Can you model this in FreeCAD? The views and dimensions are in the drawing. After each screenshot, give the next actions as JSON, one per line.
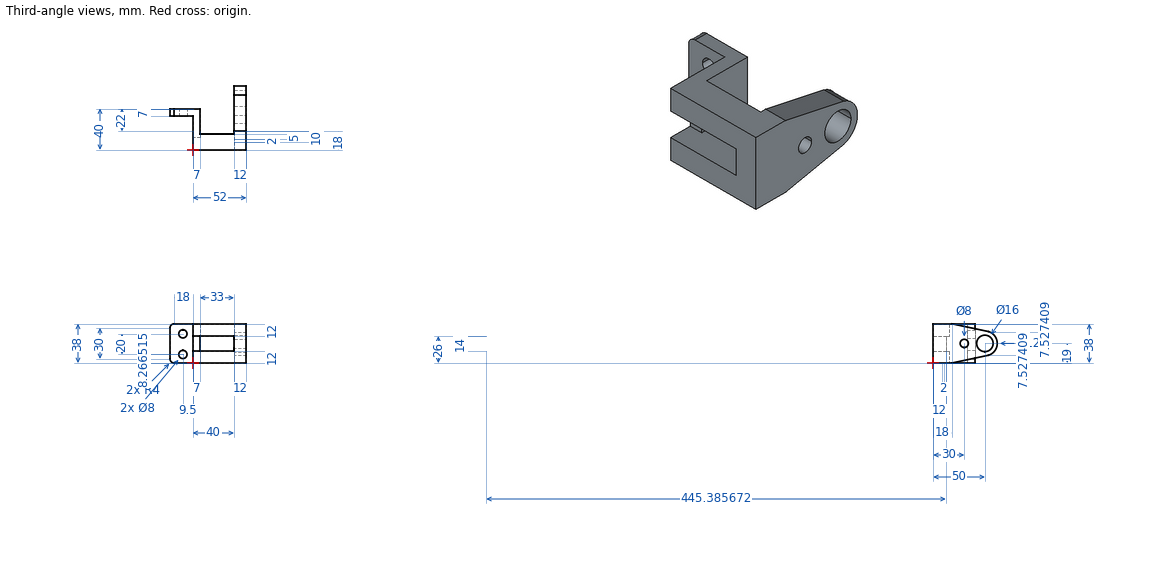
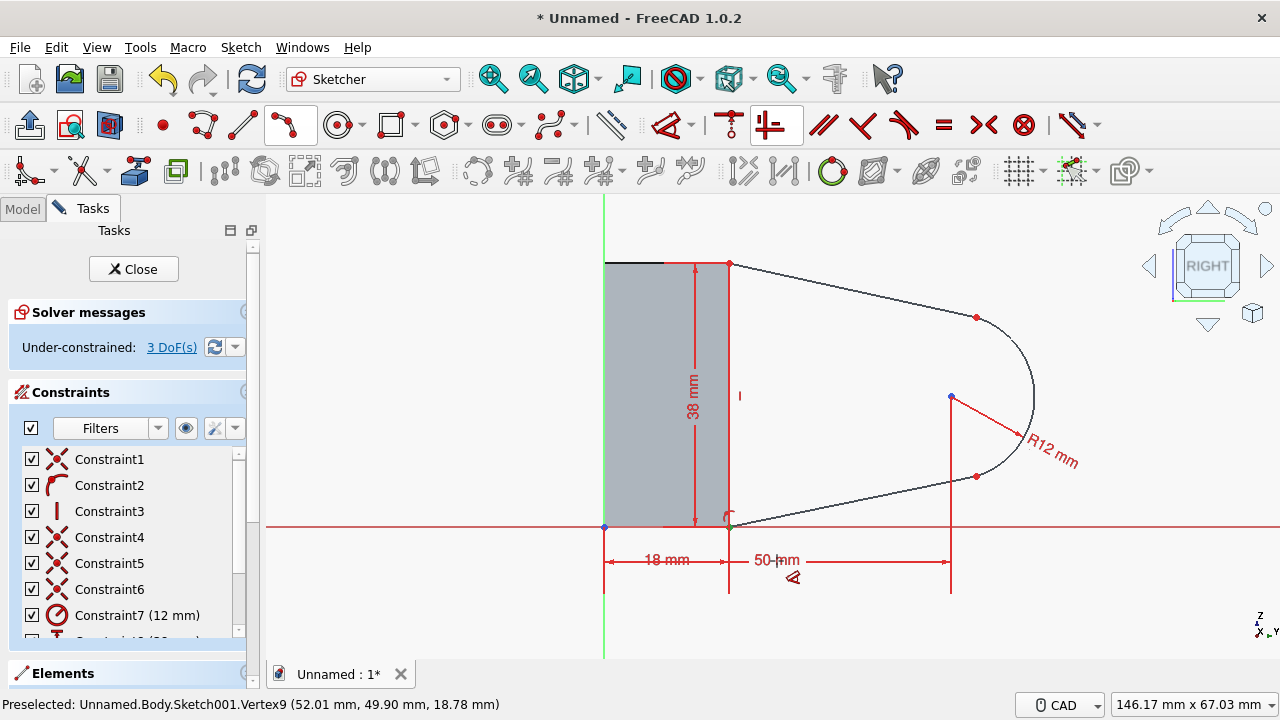
{"action": "left_click", "coordinate": [951, 397]}
{"action": "left_click", "coordinate": [570, 462]}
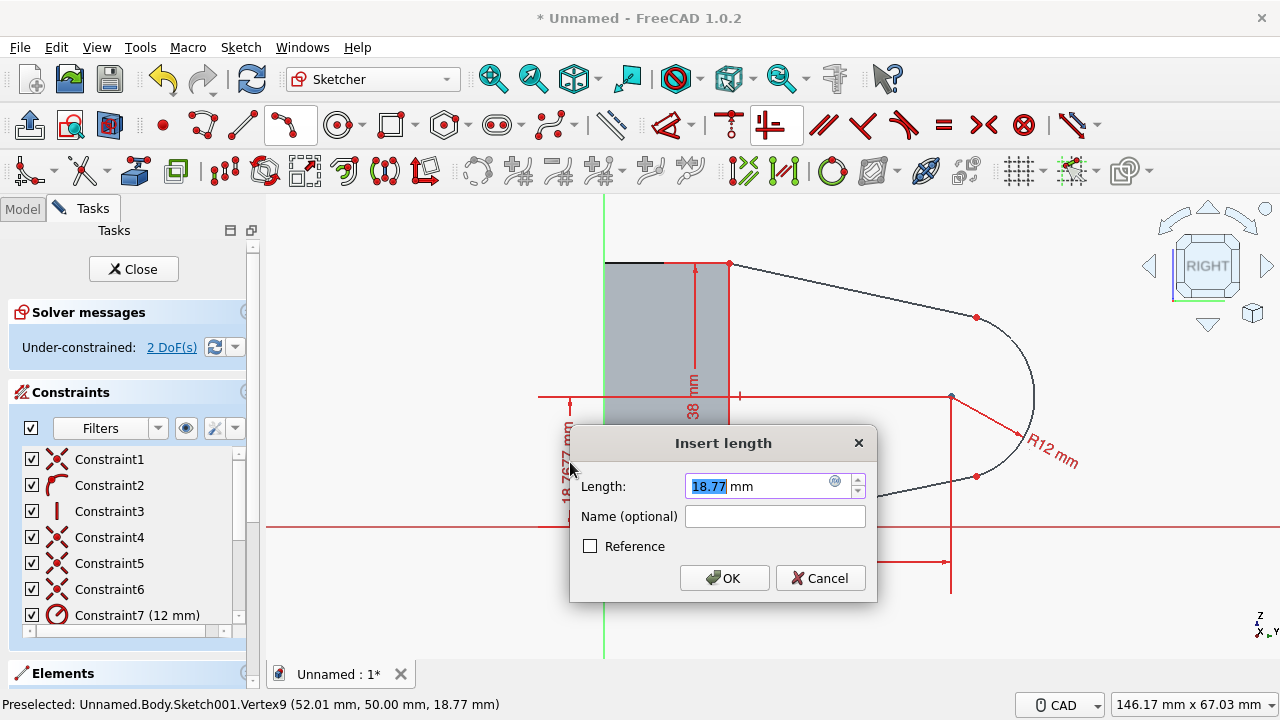
{"action": "type", "text": "19"}
{"action": "key", "text": "Return"}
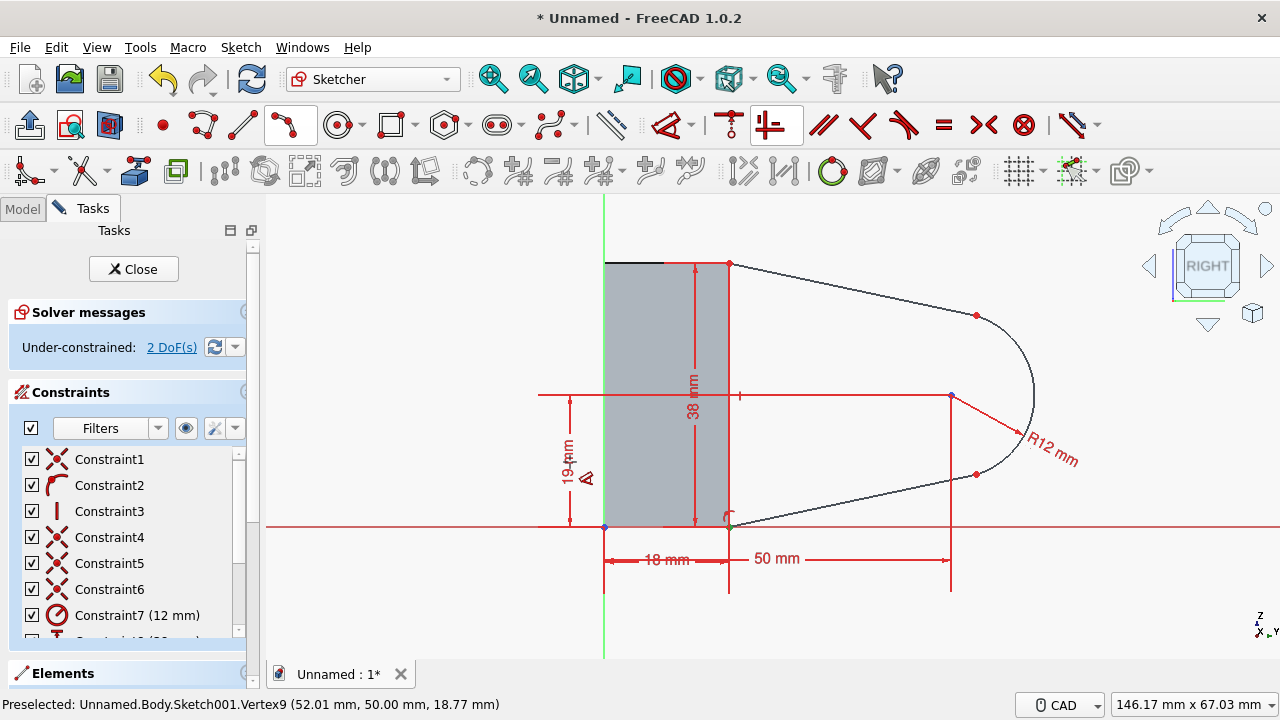
{"action": "left_click", "coordinate": [976, 475]}
{"action": "left_click", "coordinate": [570, 501]}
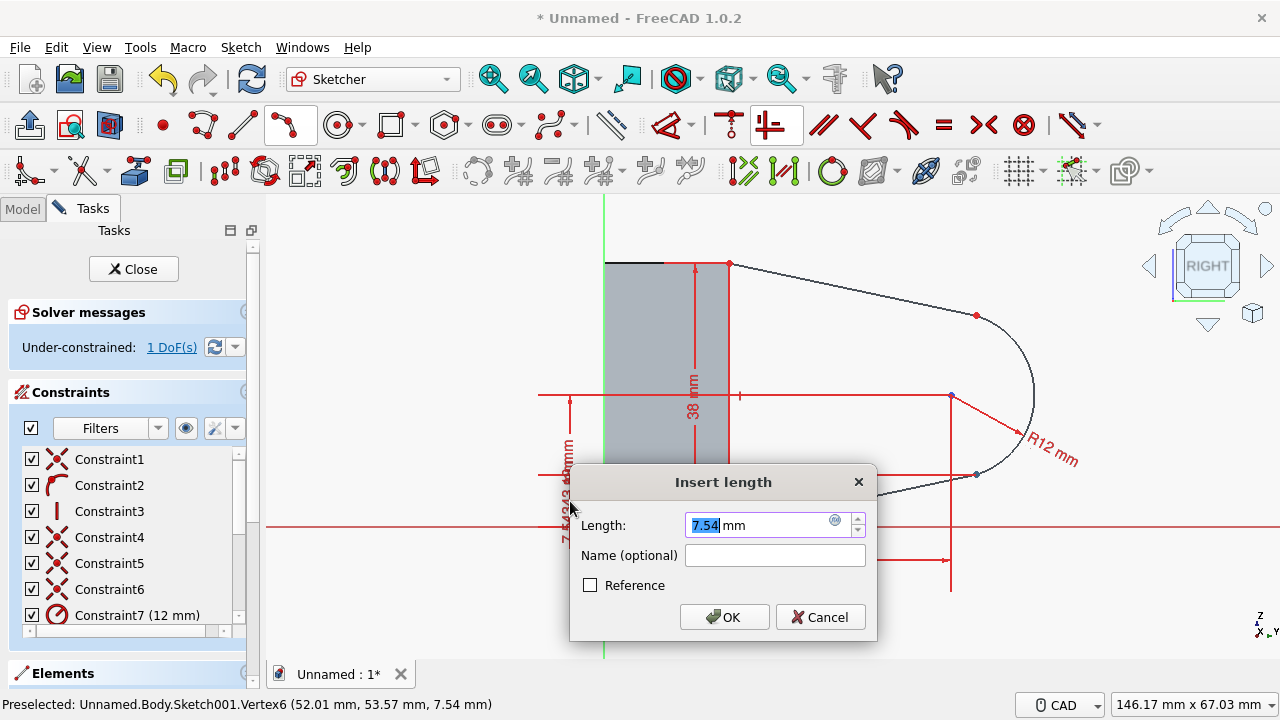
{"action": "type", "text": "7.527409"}
{"action": "key", "text": "Return"}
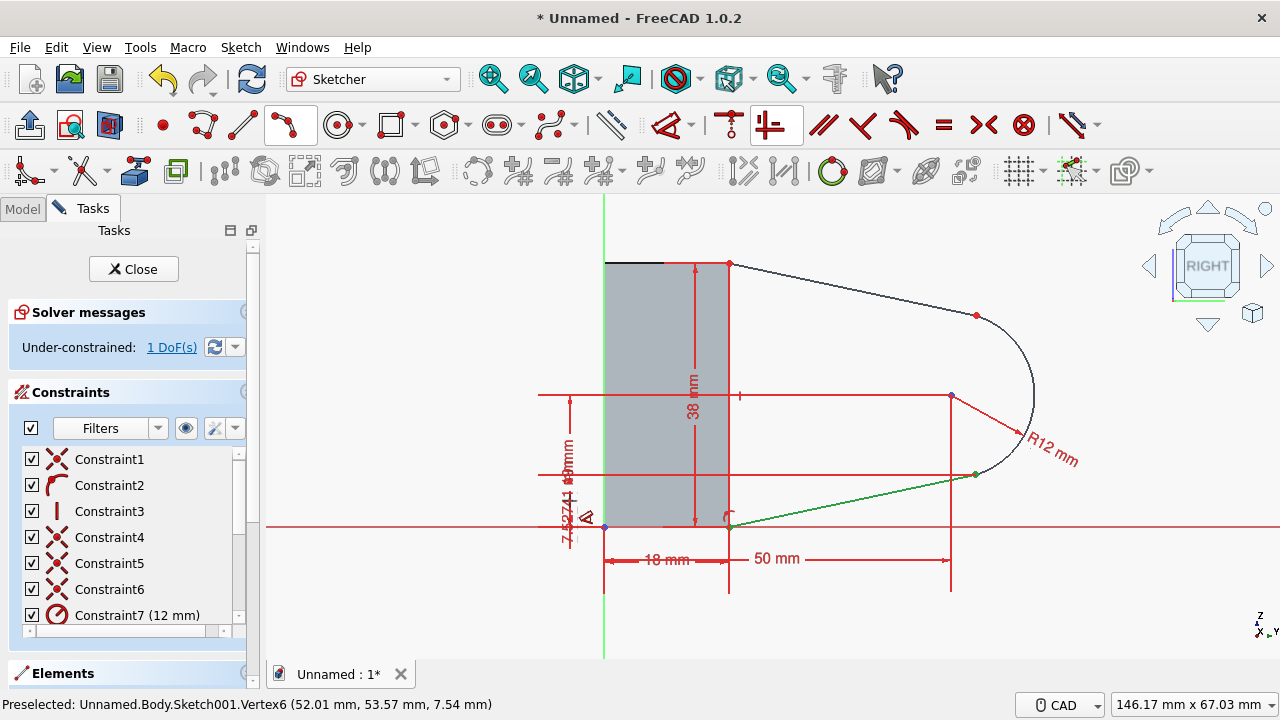
{"action": "left_click", "coordinate": [902, 300]}
{"action": "left_click", "coordinate": [1010, 290]}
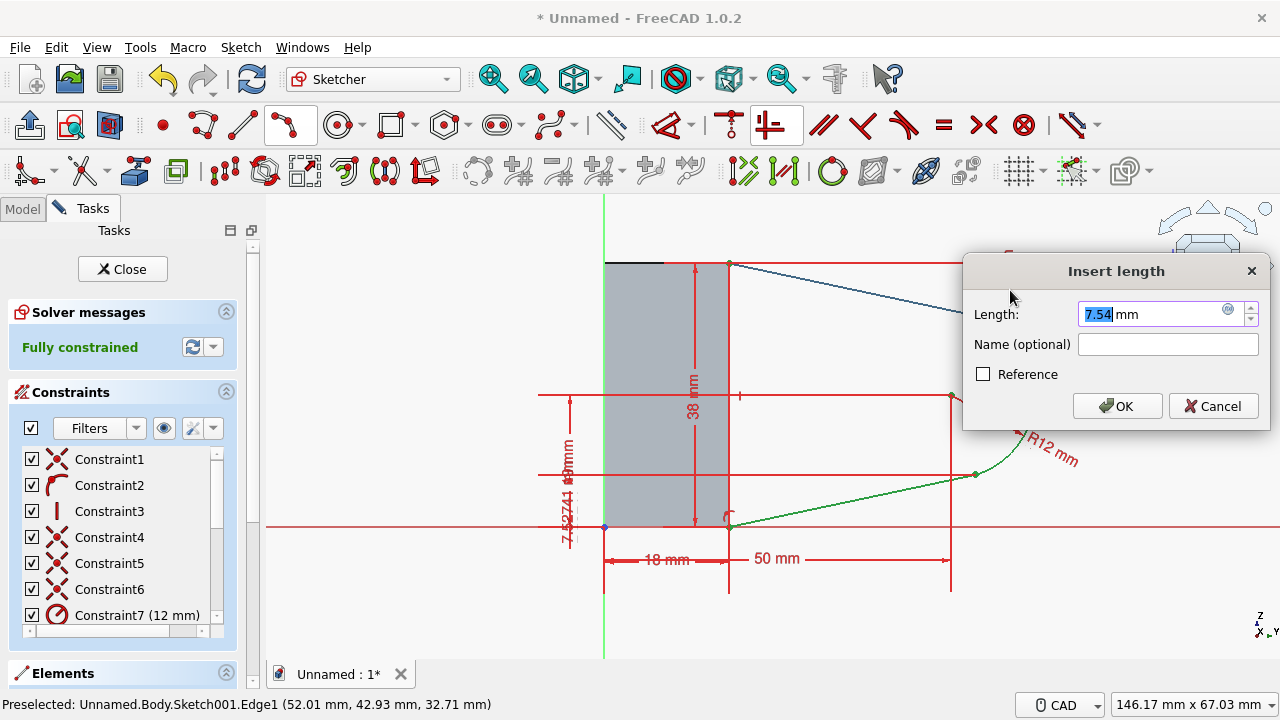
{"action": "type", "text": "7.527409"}
{"action": "key", "text": "Return"}
{"action": "key", "text": "Escape"}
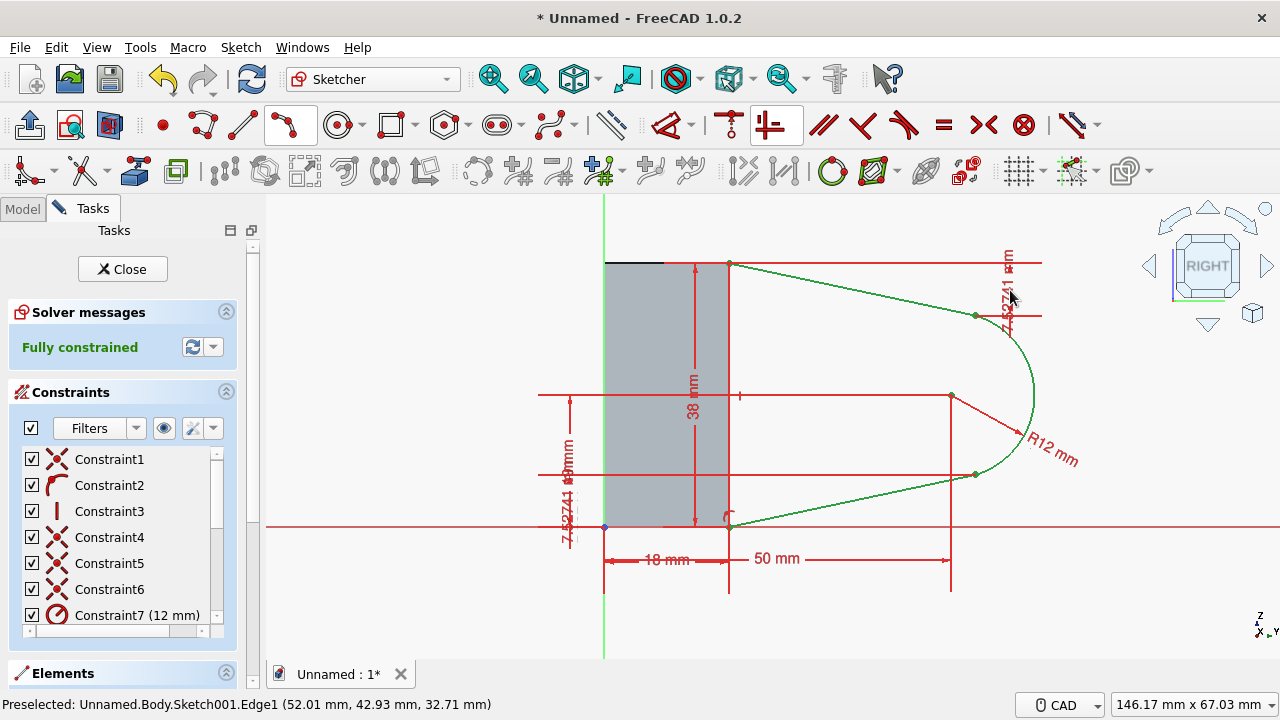
{"action": "left_click", "coordinate": [123, 269]}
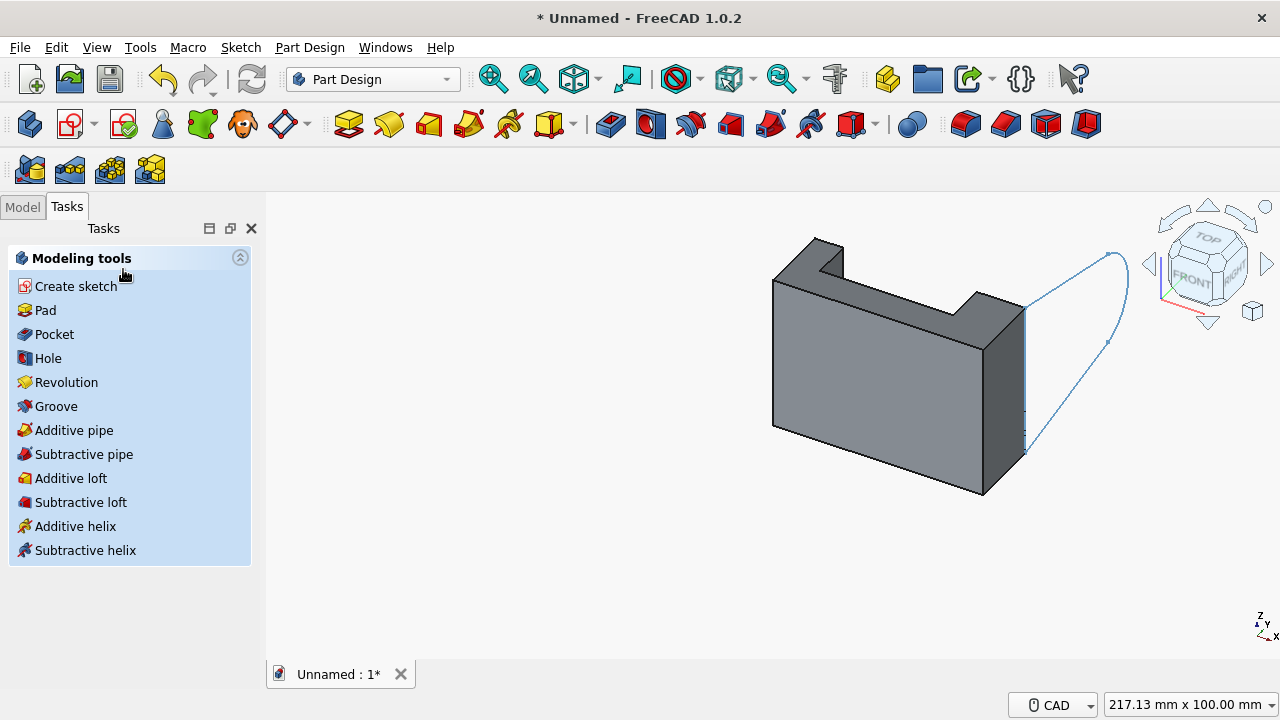
{"action": "left_click", "coordinate": [350, 124]}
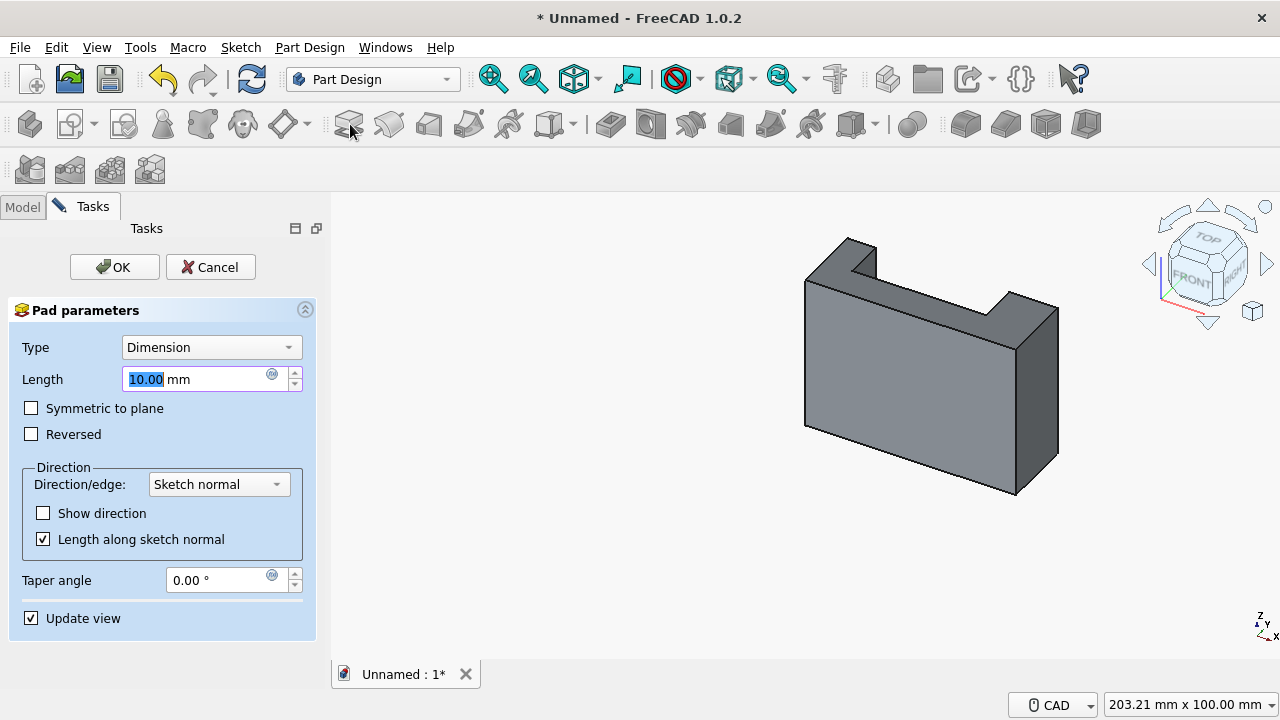
{"action": "type", "text": "12"}
{"action": "key", "text": "Tab"}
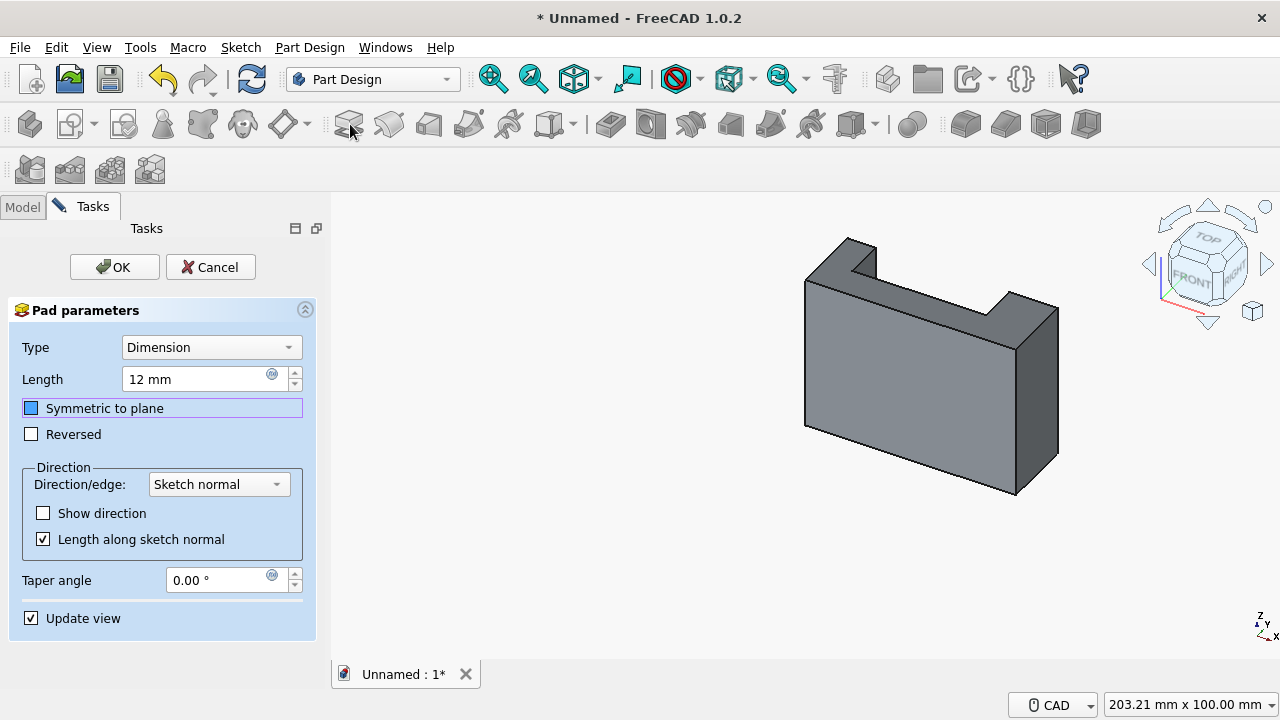
{"action": "left_click", "coordinate": [30, 434]}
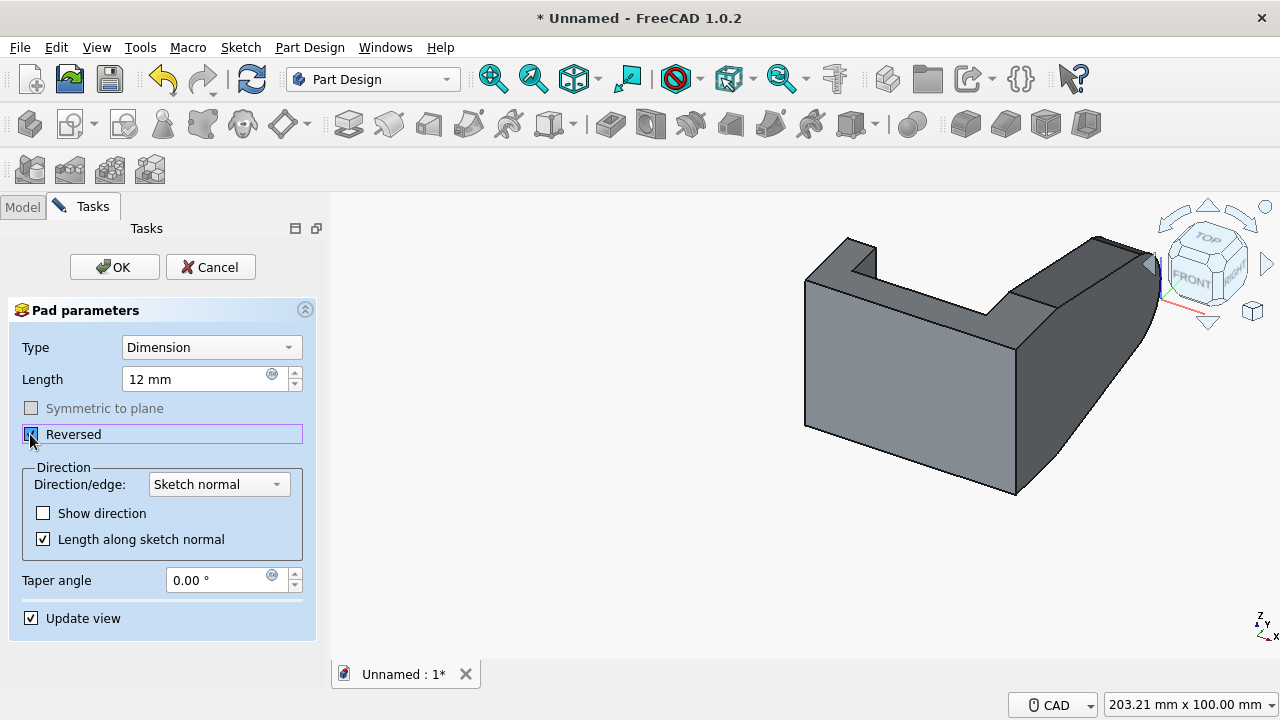
{"action": "left_click", "coordinate": [115, 267]}